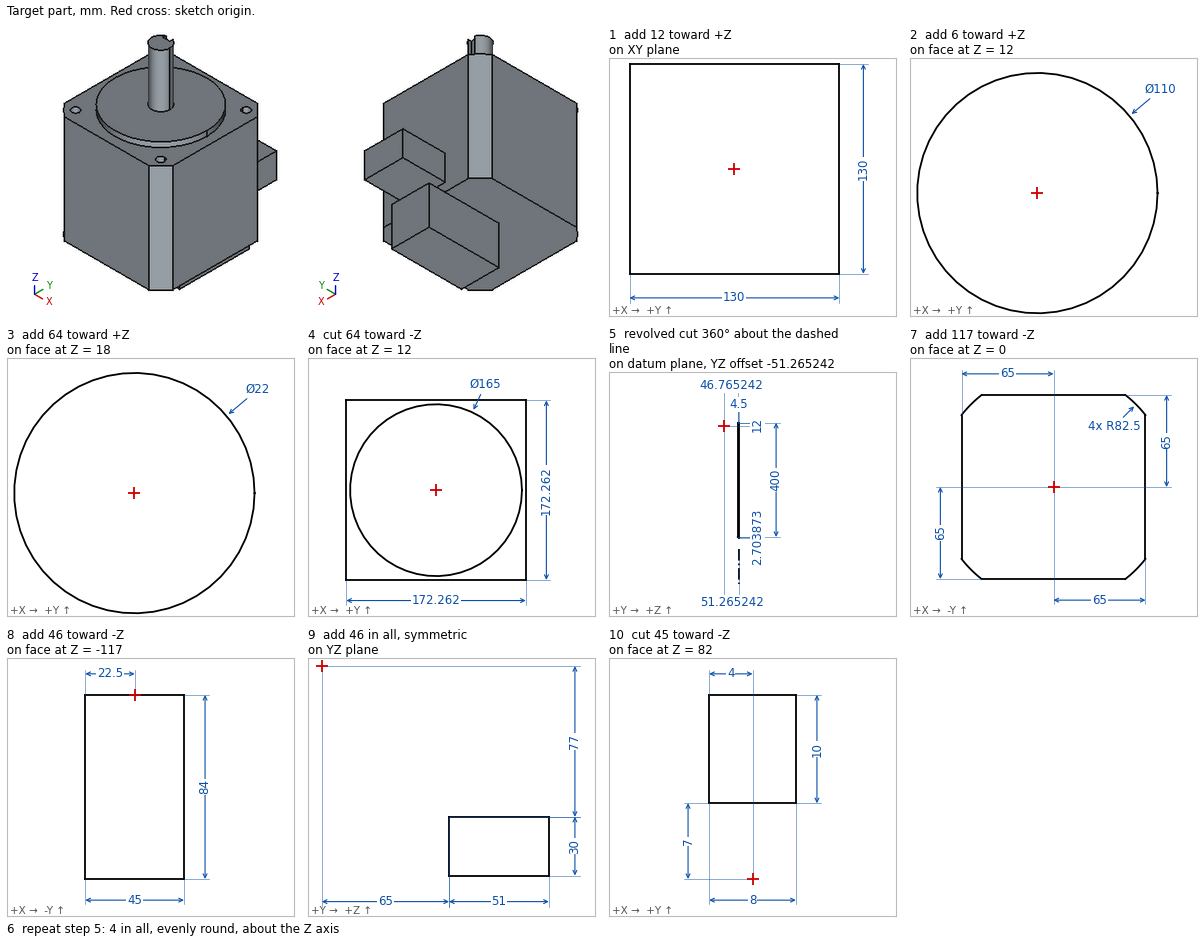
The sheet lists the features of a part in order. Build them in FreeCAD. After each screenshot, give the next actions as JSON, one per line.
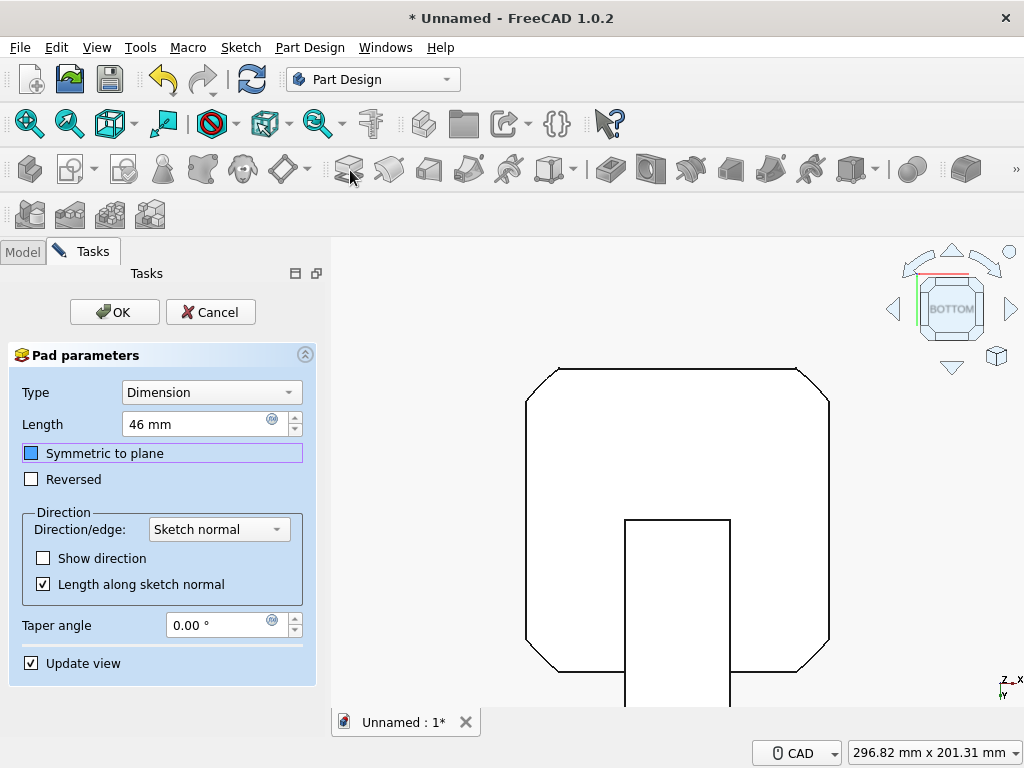
{"action": "left_click", "coordinate": [115, 312]}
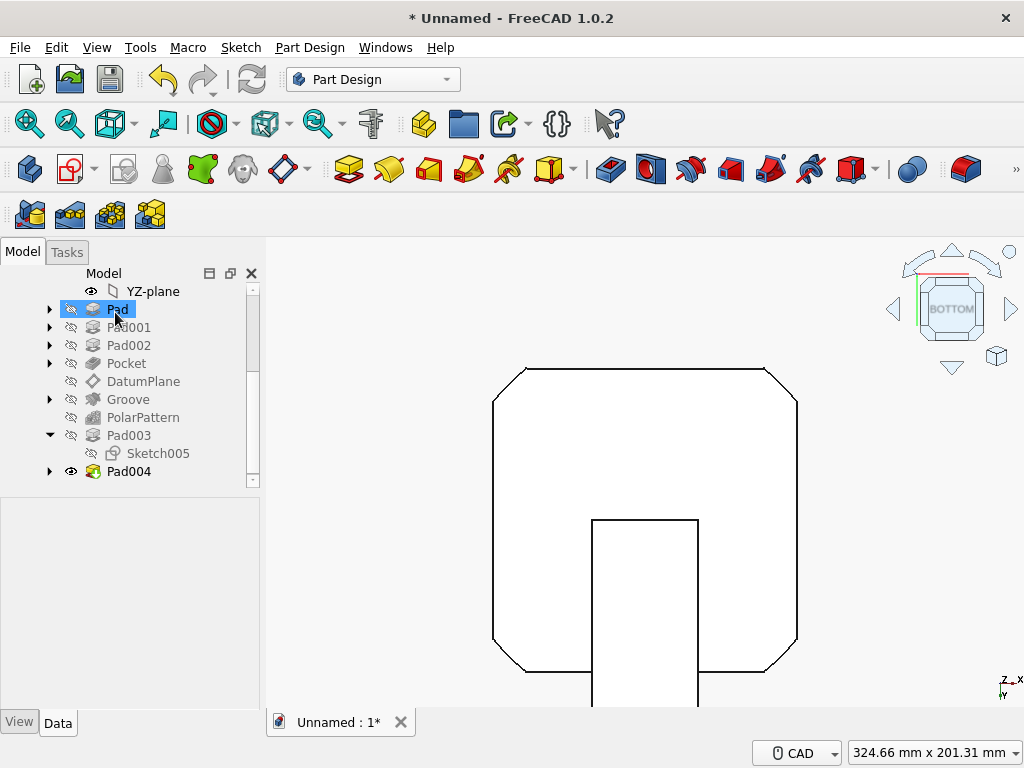
{"action": "left_click", "coordinate": [30, 124]}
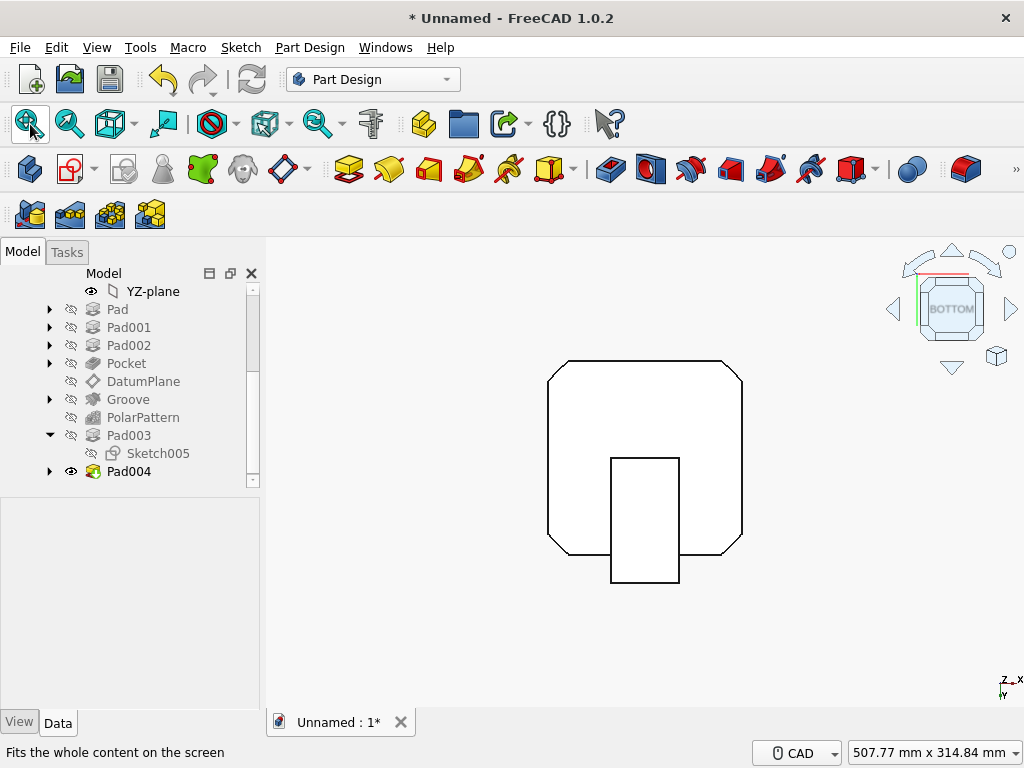
{"action": "left_click", "coordinate": [70, 170]}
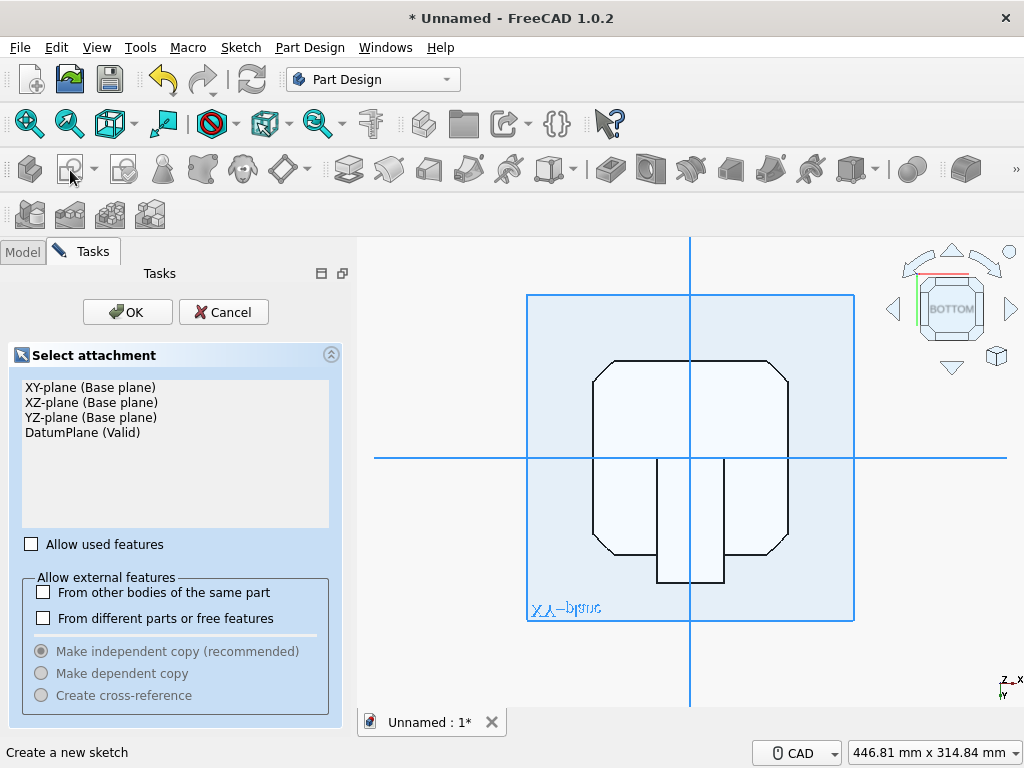
{"action": "left_click", "coordinate": [82, 418]}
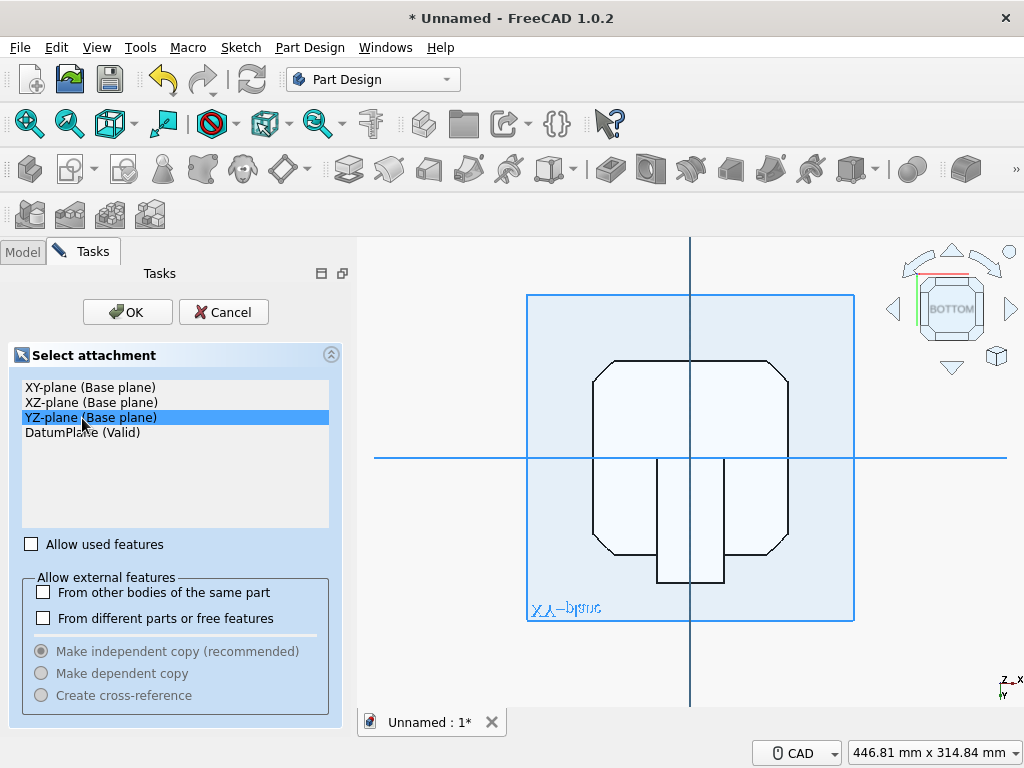
{"action": "left_click", "coordinate": [128, 312]}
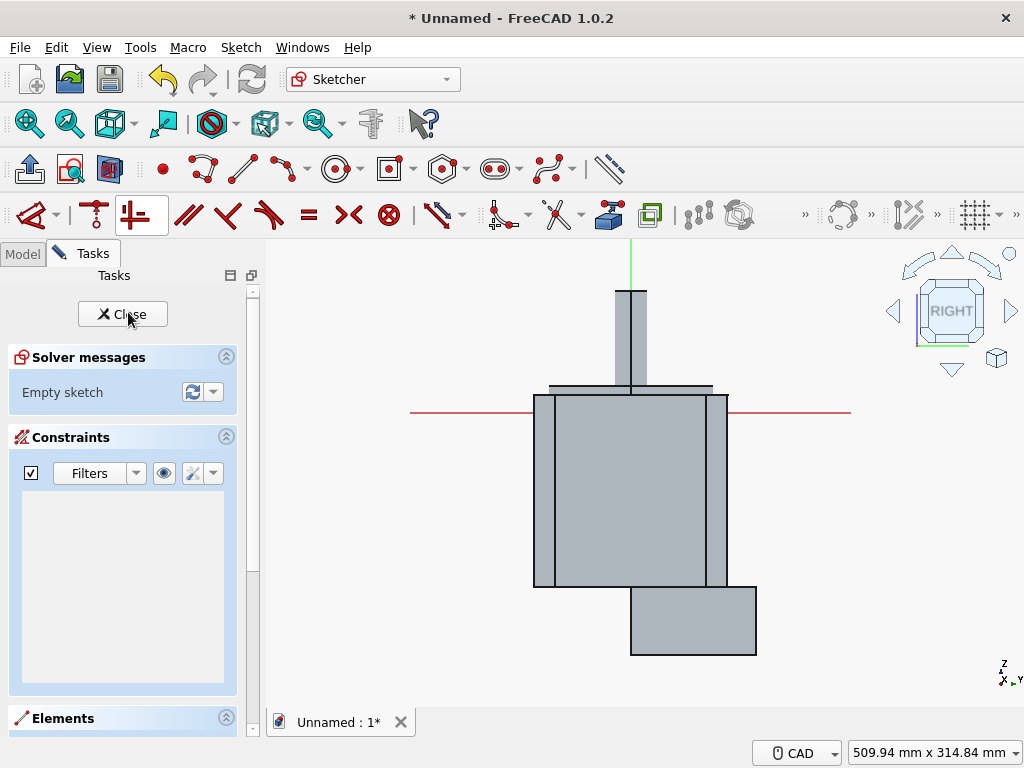
{"action": "key", "text": "q s"}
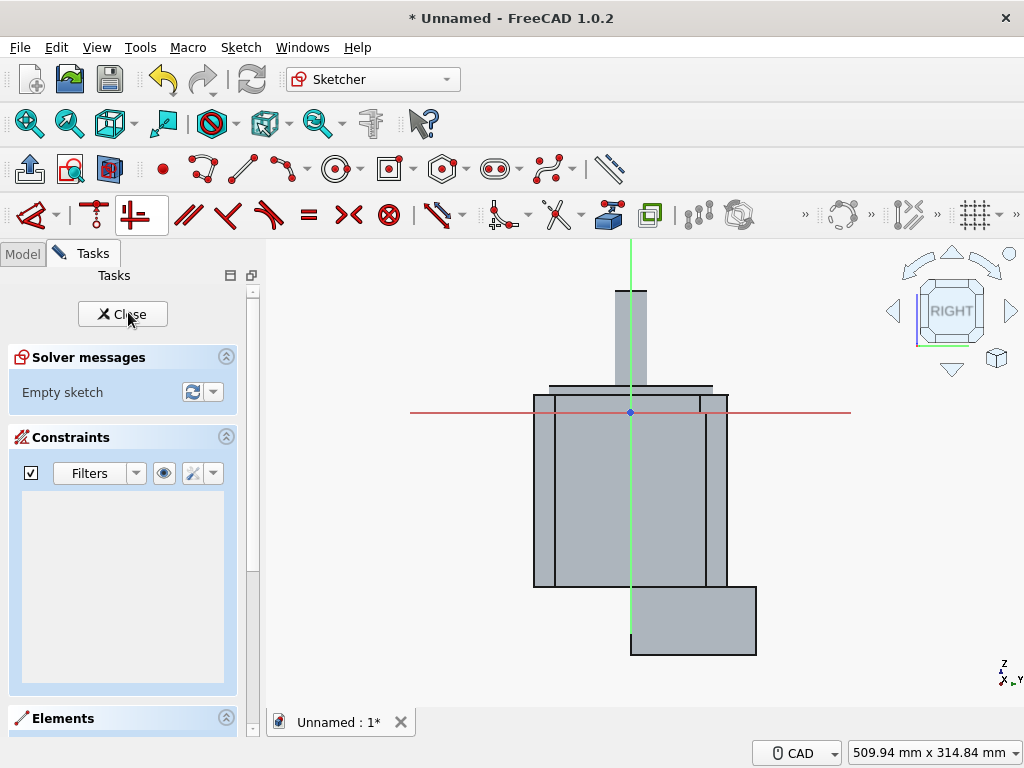
{"action": "scroll", "coordinate": [859, 516], "scroll_direction": "up", "scroll_amount": 3}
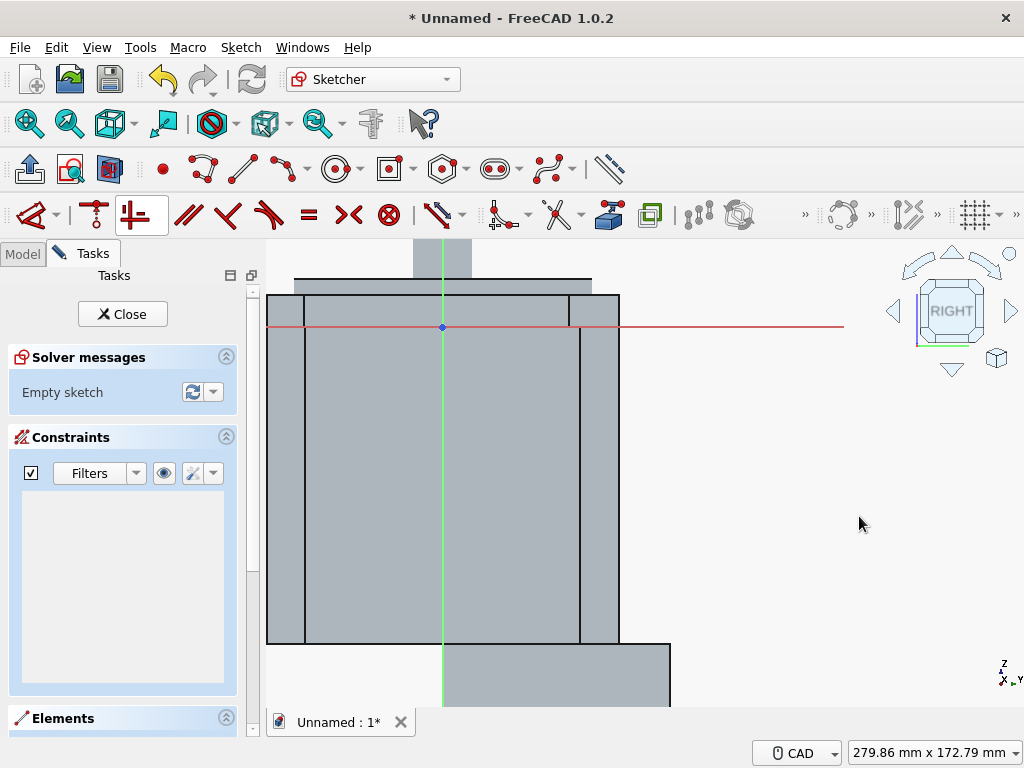
{"action": "key", "text": "g r"}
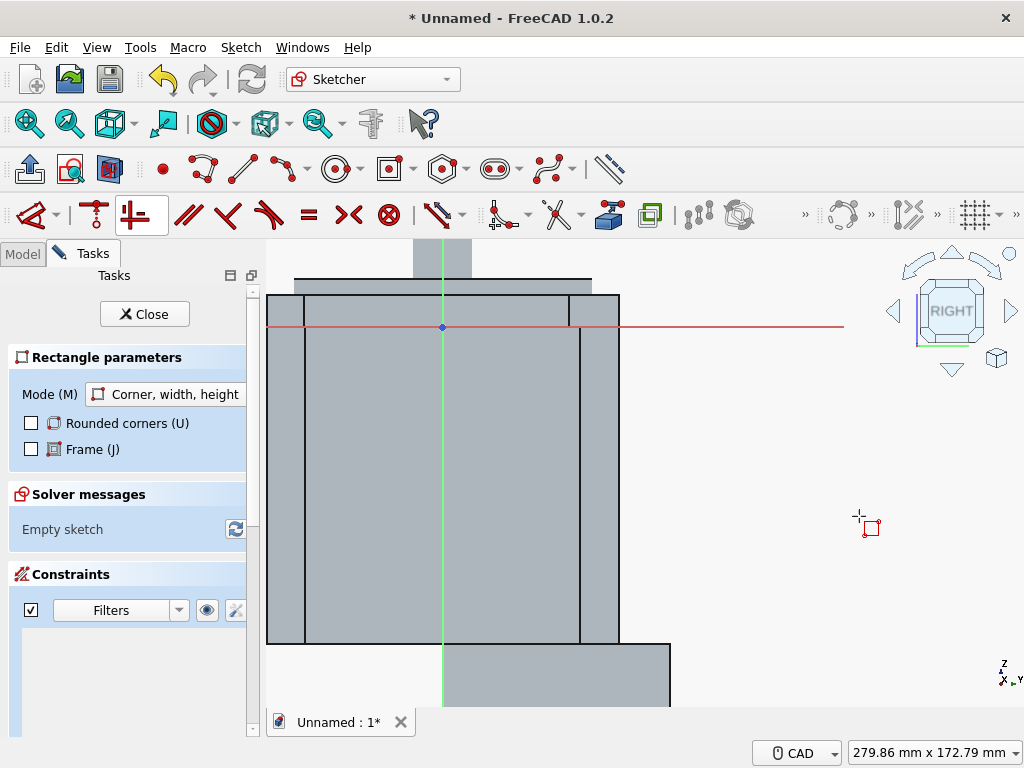
{"action": "left_click", "coordinate": [619, 536]}
{"action": "mouse_move", "coordinate": [757, 617]}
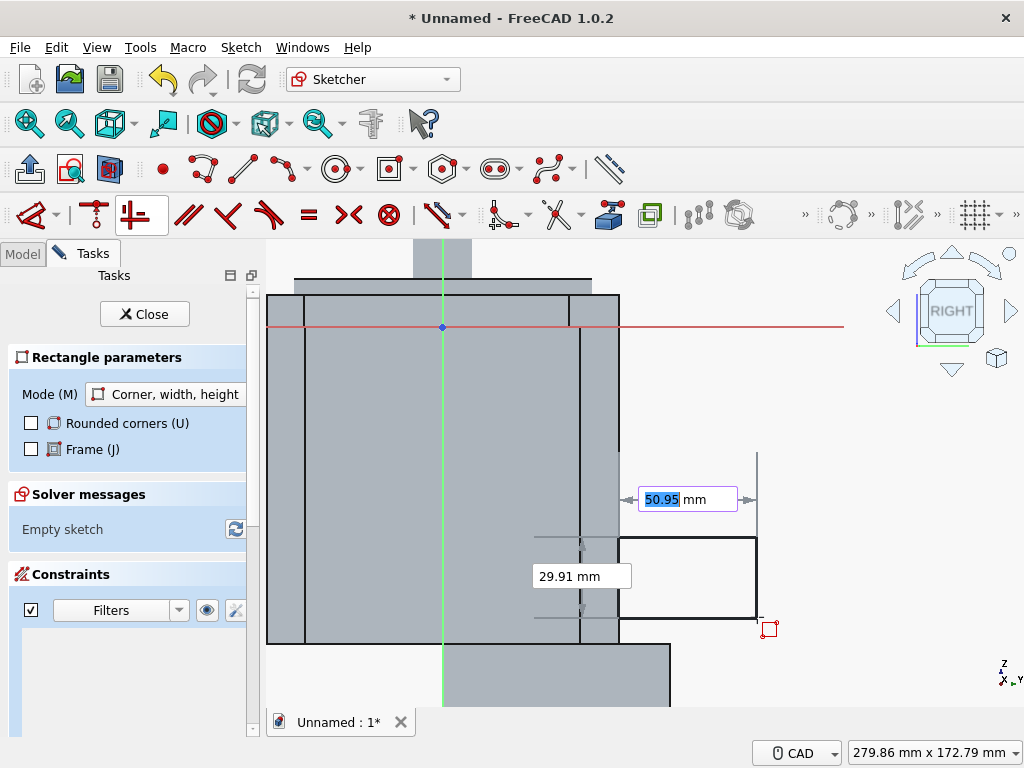
{"action": "type", "text": "51"}
{"action": "key", "text": "Tab"}
{"action": "type", "text": "30"}
{"action": "key", "text": "Return"}
{"action": "key", "text": "Escape"}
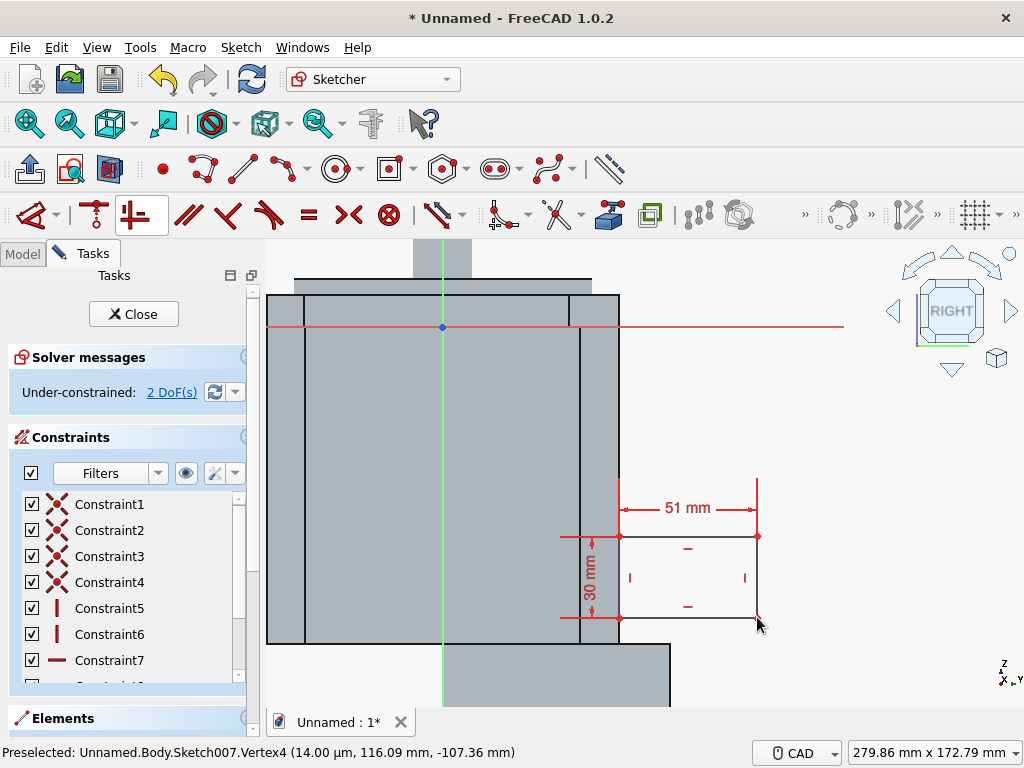
{"action": "left_click", "coordinate": [32, 216]}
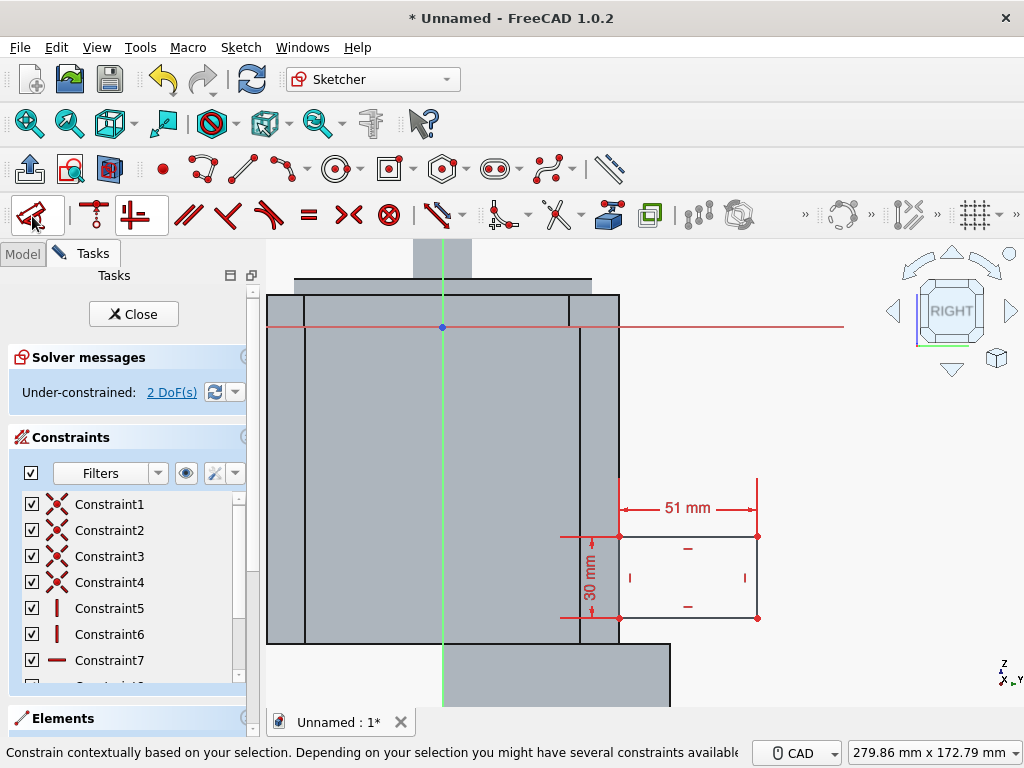
{"action": "left_click", "coordinate": [619, 537]}
{"action": "left_click", "coordinate": [531, 293]}